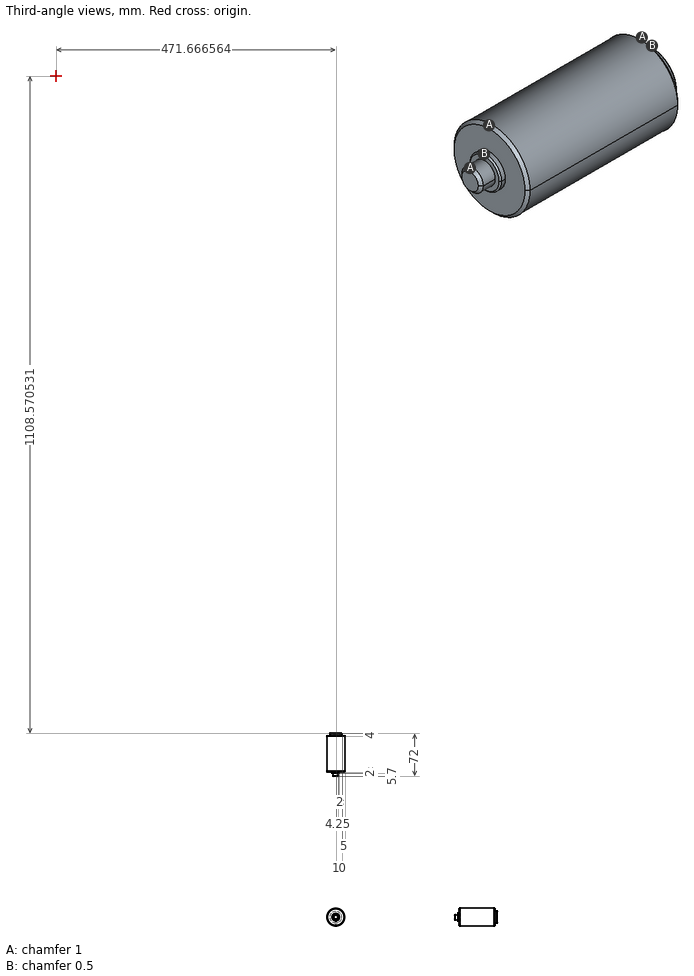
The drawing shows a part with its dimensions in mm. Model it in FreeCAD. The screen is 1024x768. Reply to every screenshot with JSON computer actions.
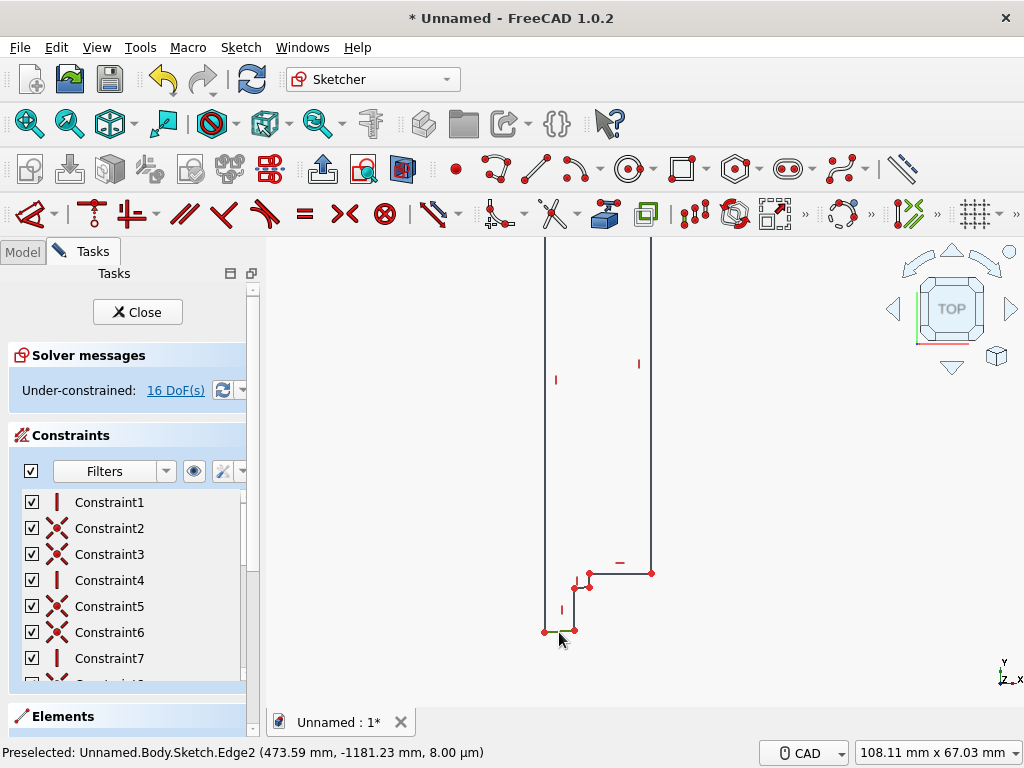
{"action": "key", "text": "h"}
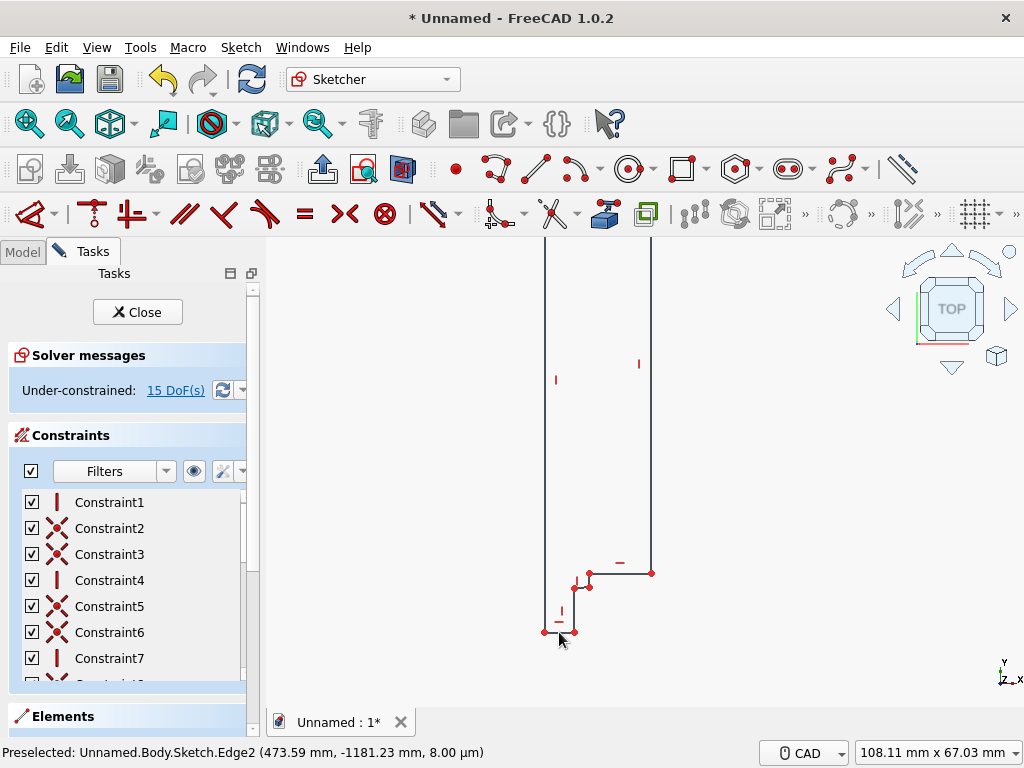
{"action": "scroll", "coordinate": [582, 588], "scroll_direction": "up", "scroll_amount": 4}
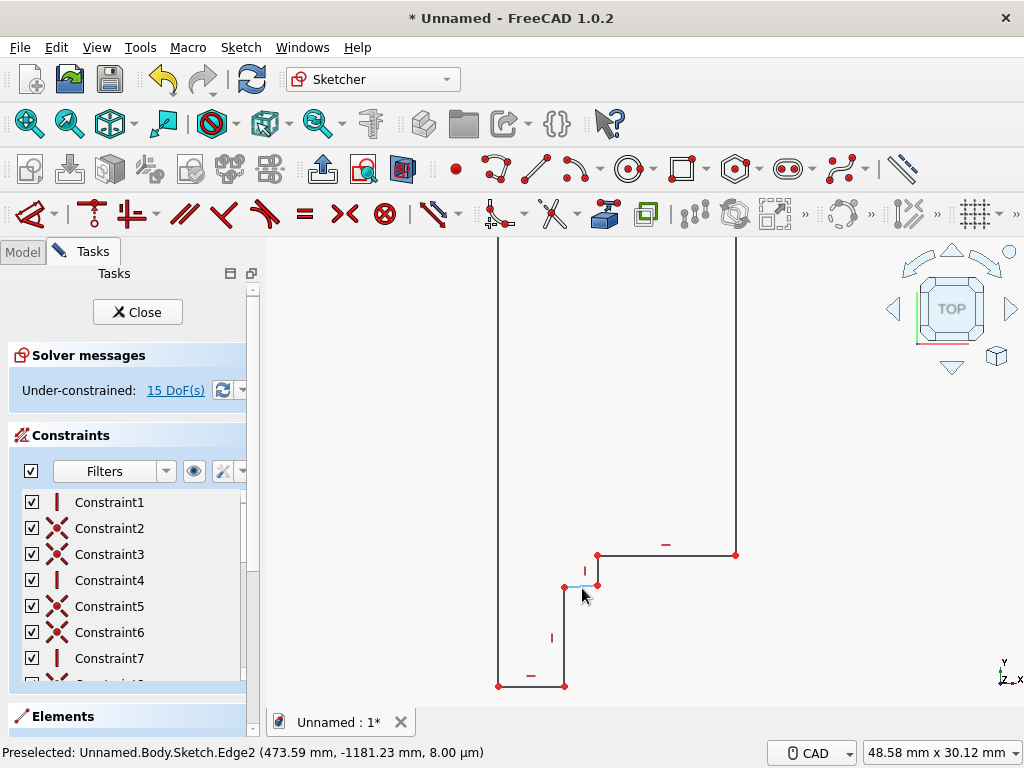
{"action": "left_click", "coordinate": [581, 586]}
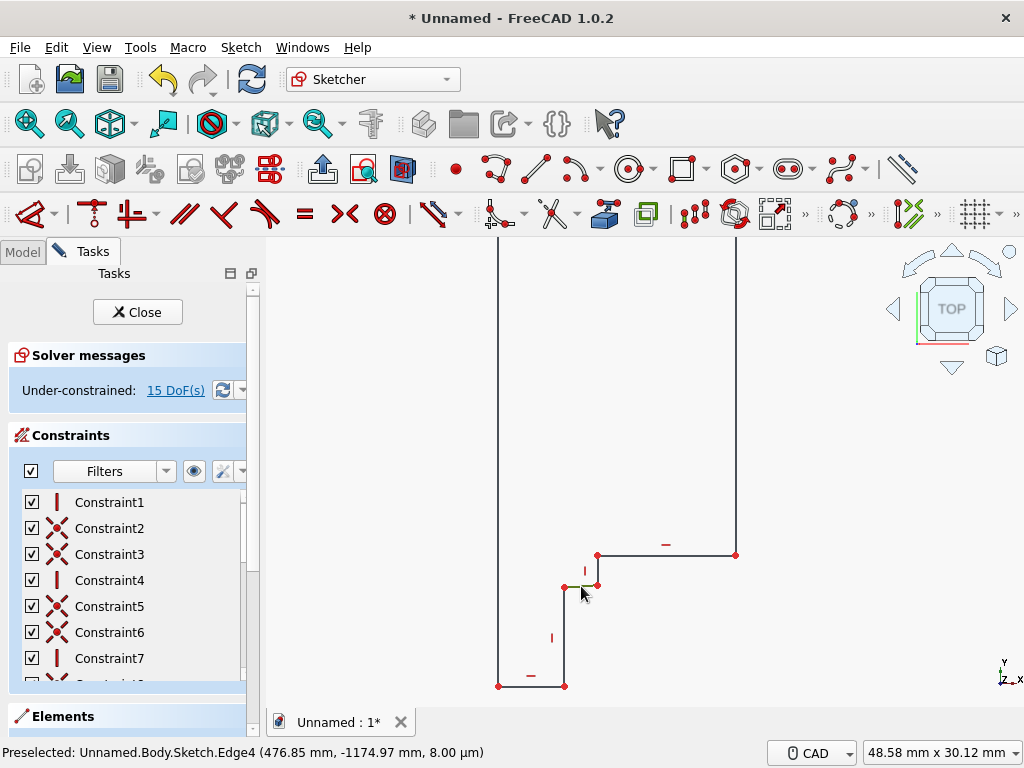
{"action": "left_click", "coordinate": [158, 214]}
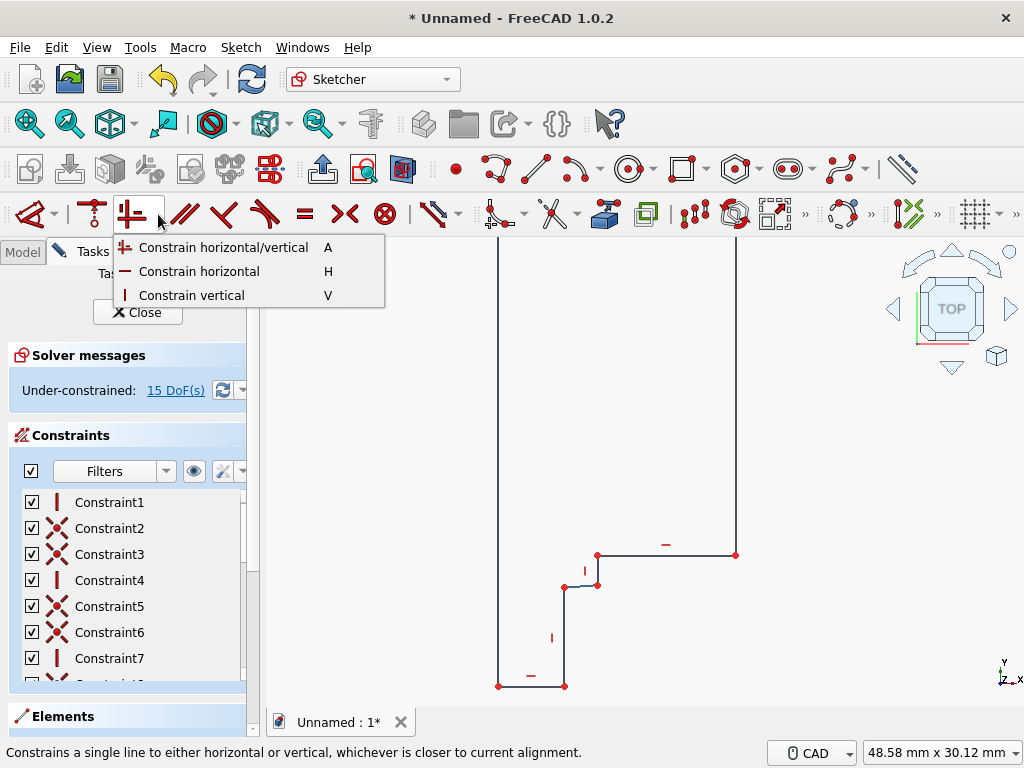
{"action": "left_click", "coordinate": [249, 271]}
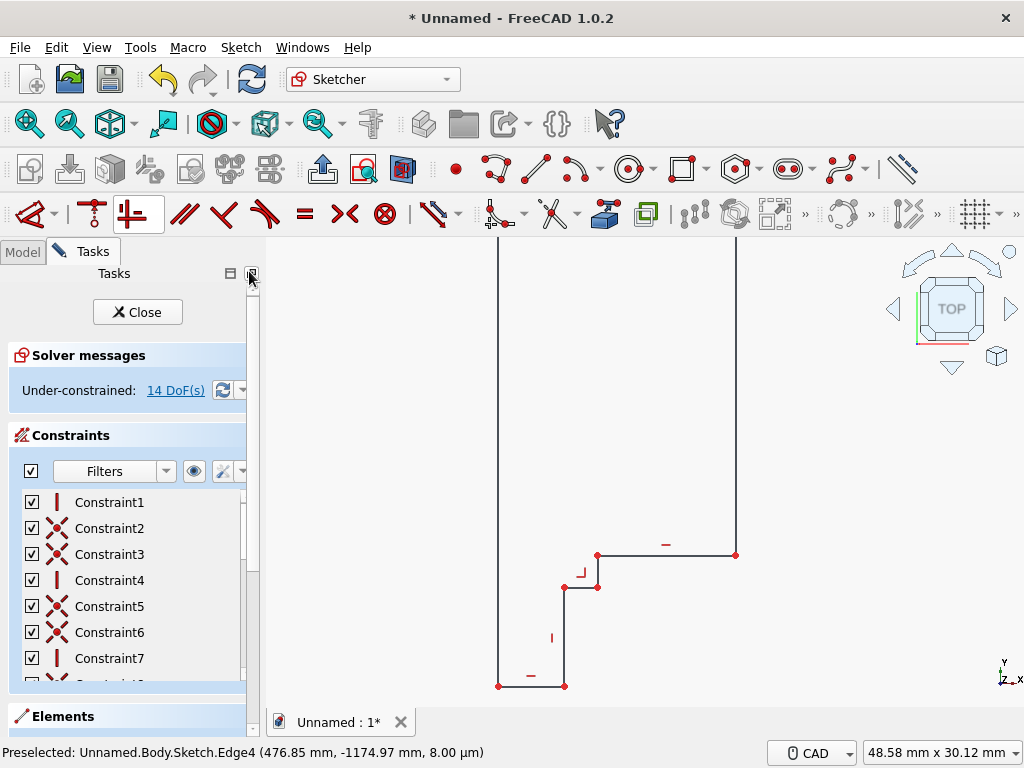
{"action": "scroll", "coordinate": [566, 620], "scroll_direction": "down", "scroll_amount": 8}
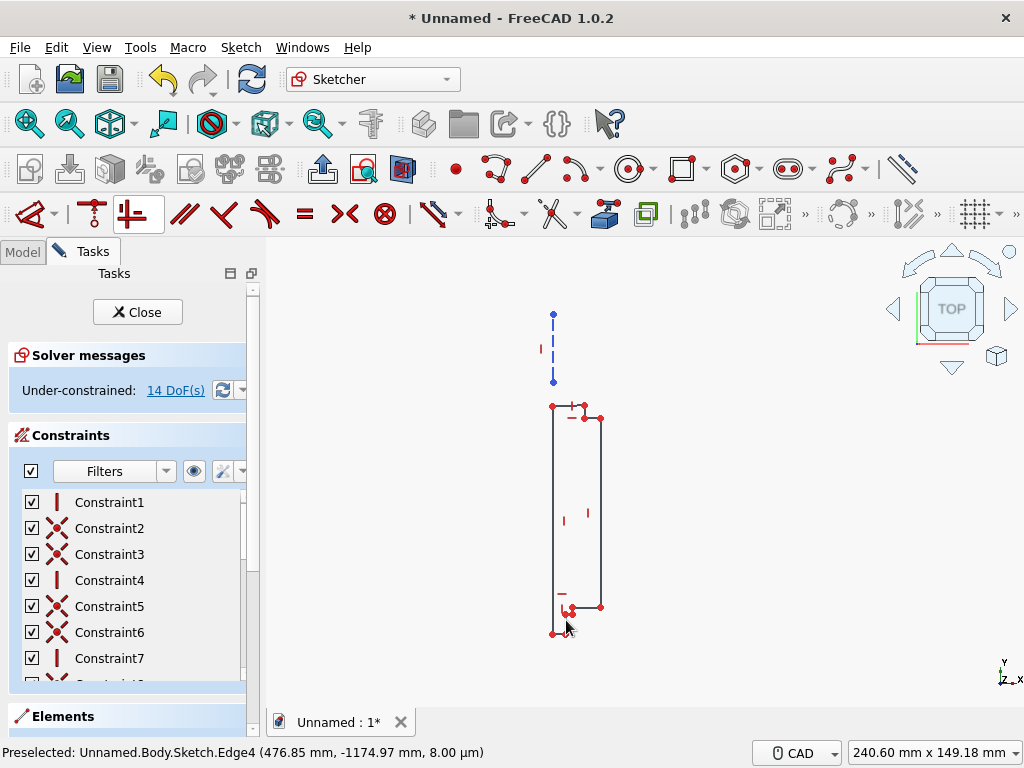
{"action": "scroll", "coordinate": [575, 406], "scroll_direction": "up", "scroll_amount": 2}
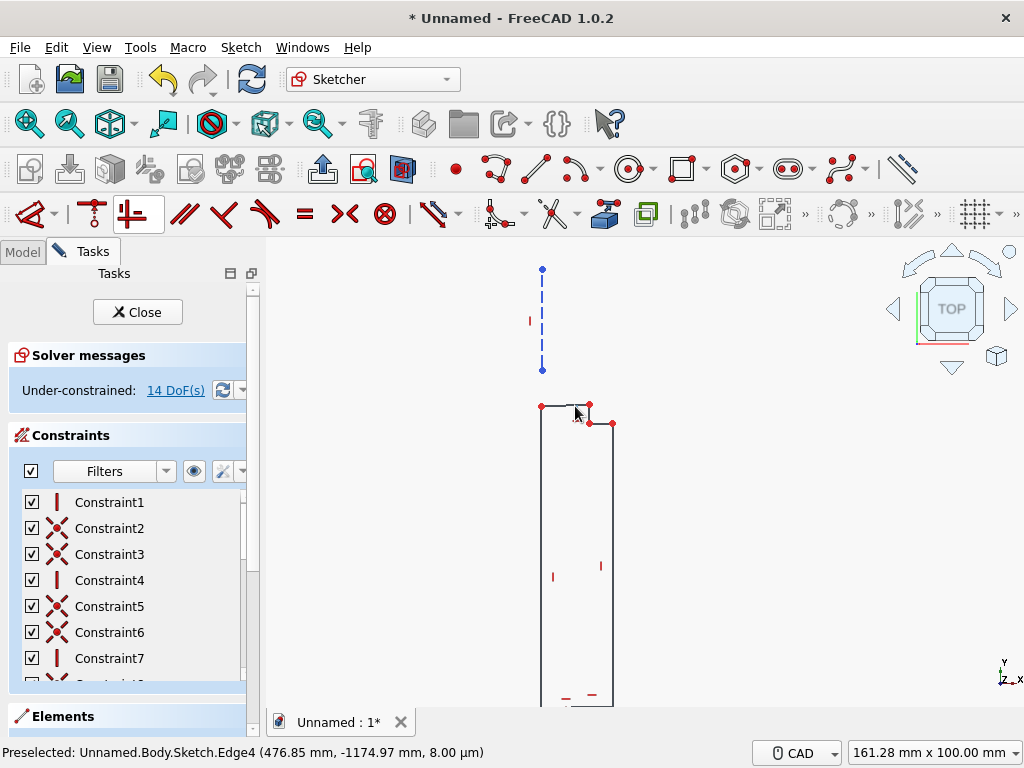
{"action": "left_click", "coordinate": [556, 406]}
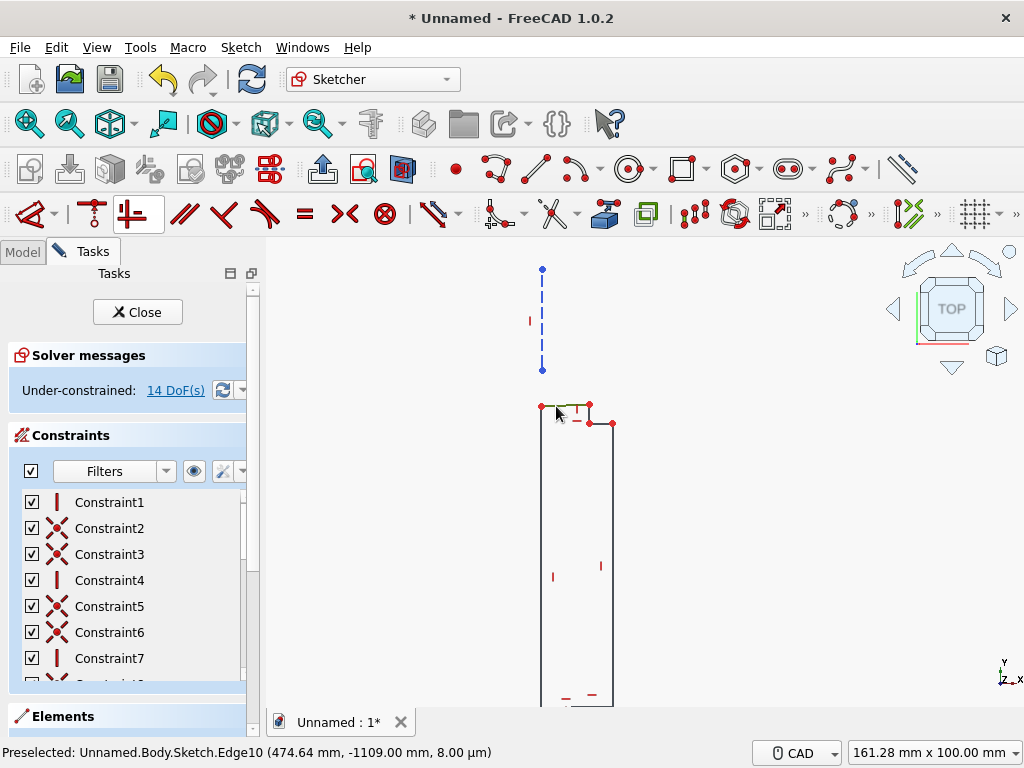
{"action": "left_click", "coordinate": [158, 214]}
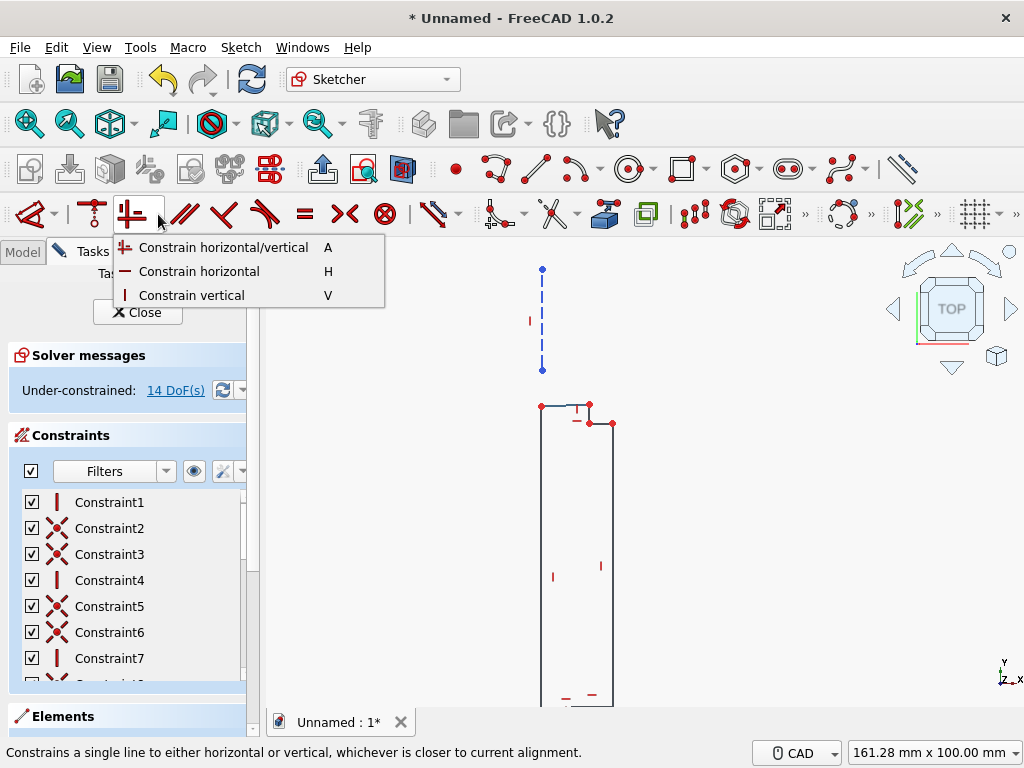
{"action": "left_click", "coordinate": [249, 271]}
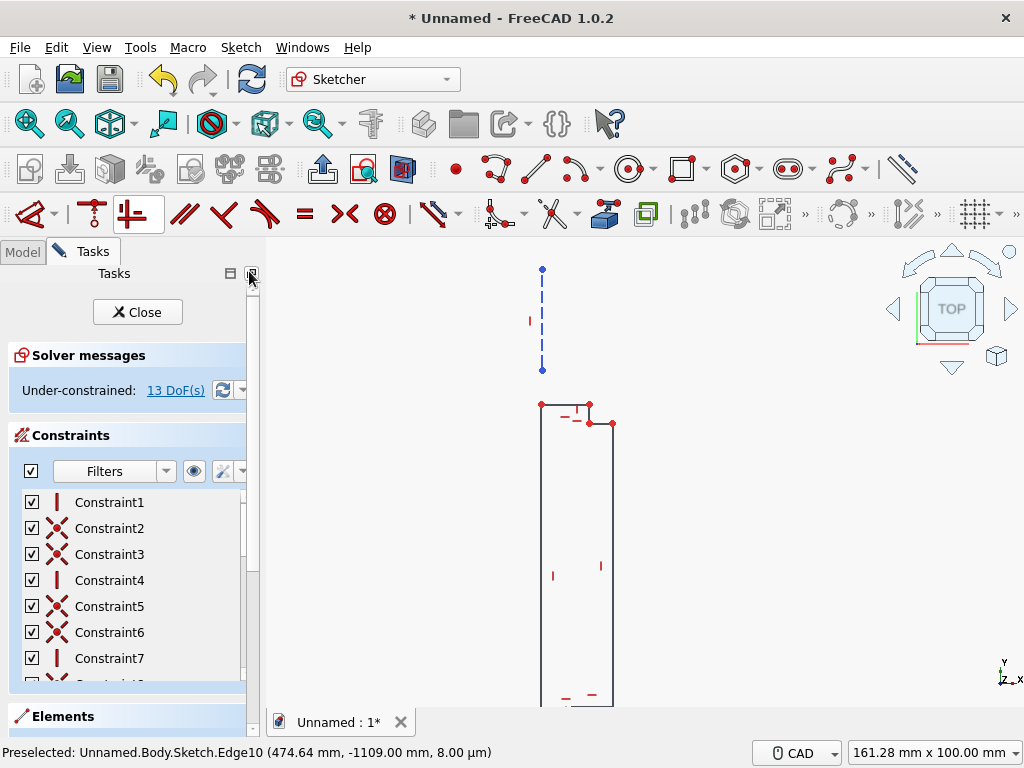
{"action": "key", "text": "d"}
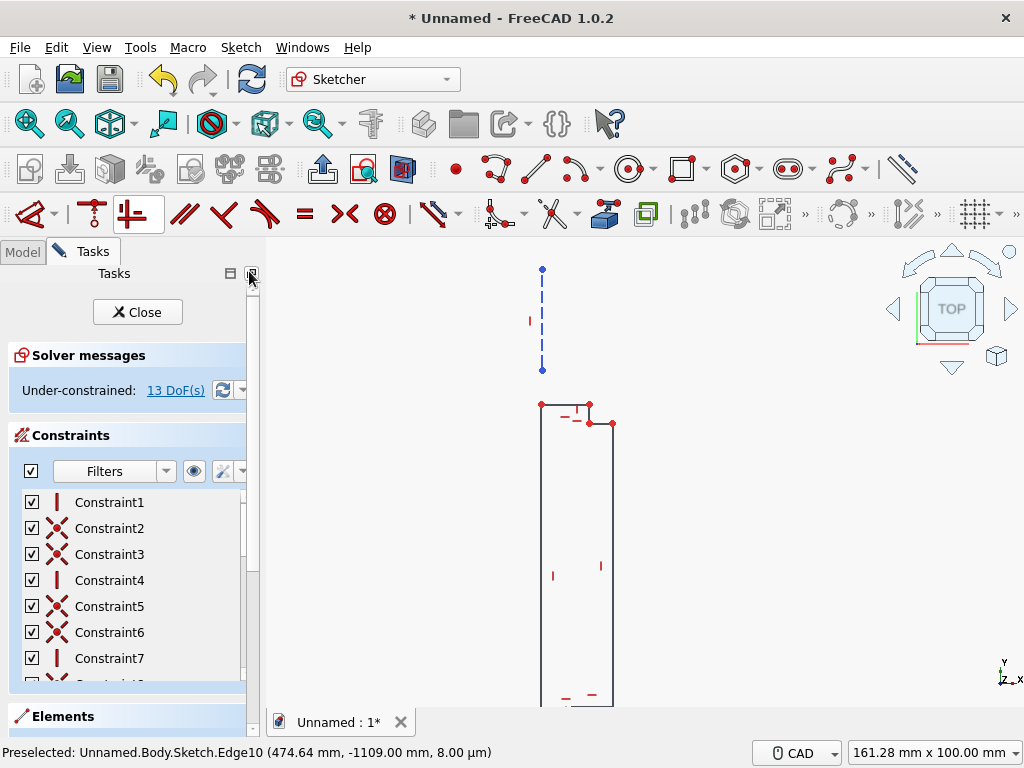
{"action": "scroll", "coordinate": [575, 404], "scroll_direction": "down", "scroll_amount": 2}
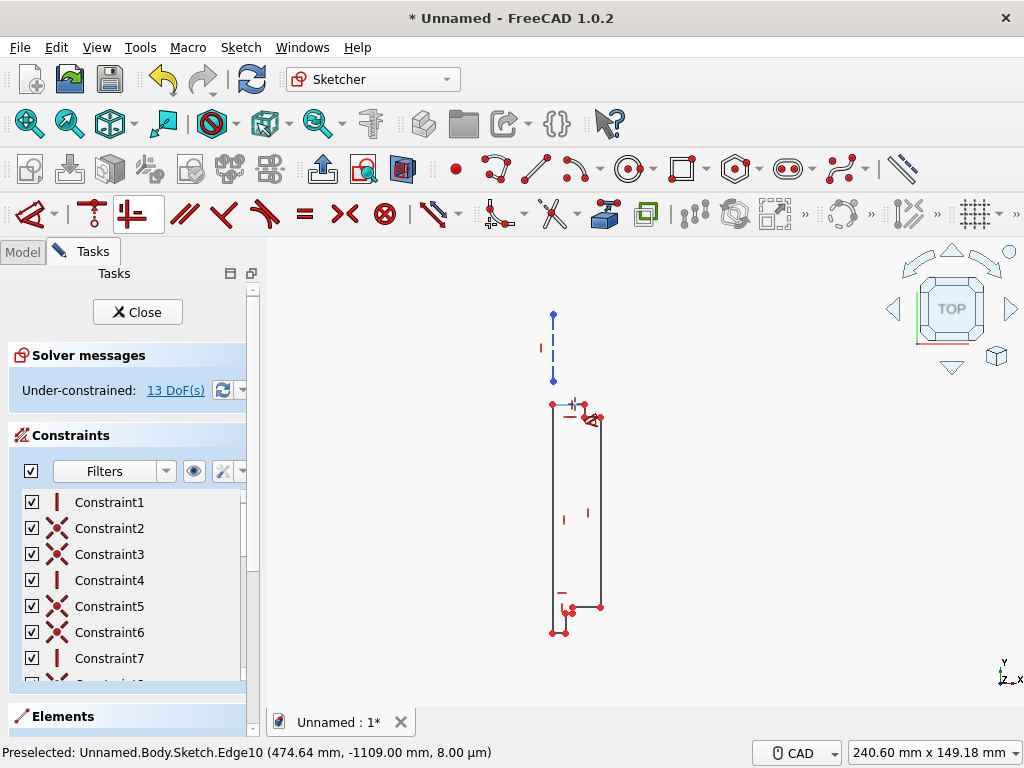
{"action": "scroll", "coordinate": [569, 613], "scroll_direction": "up", "scroll_amount": 10}